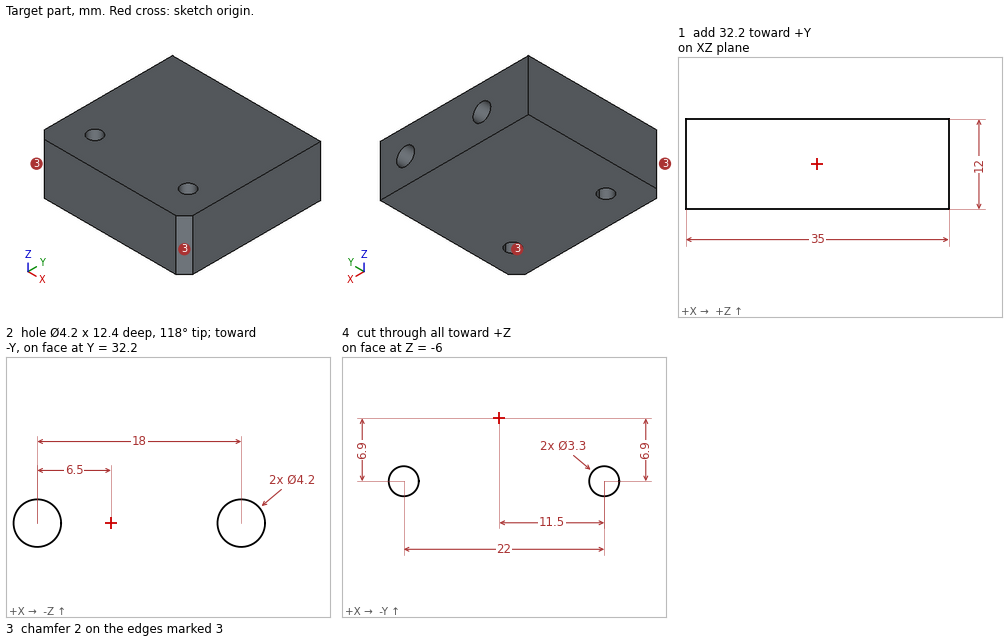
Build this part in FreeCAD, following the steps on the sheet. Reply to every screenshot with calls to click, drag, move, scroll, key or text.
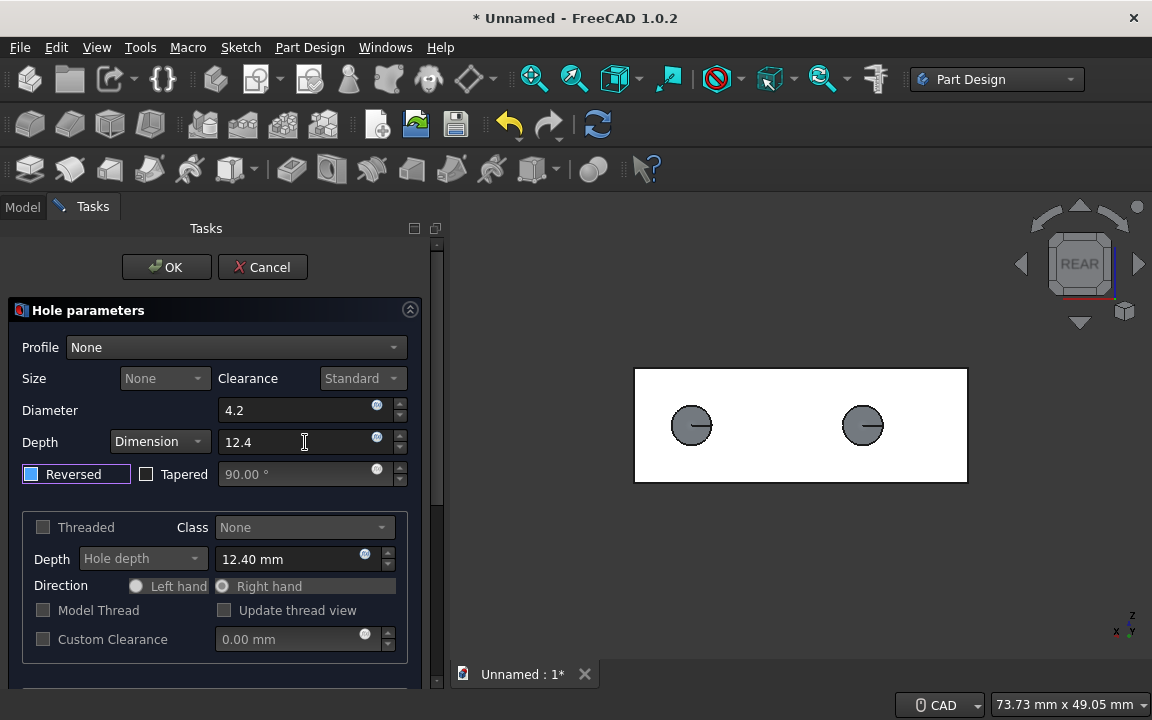
click(167, 267)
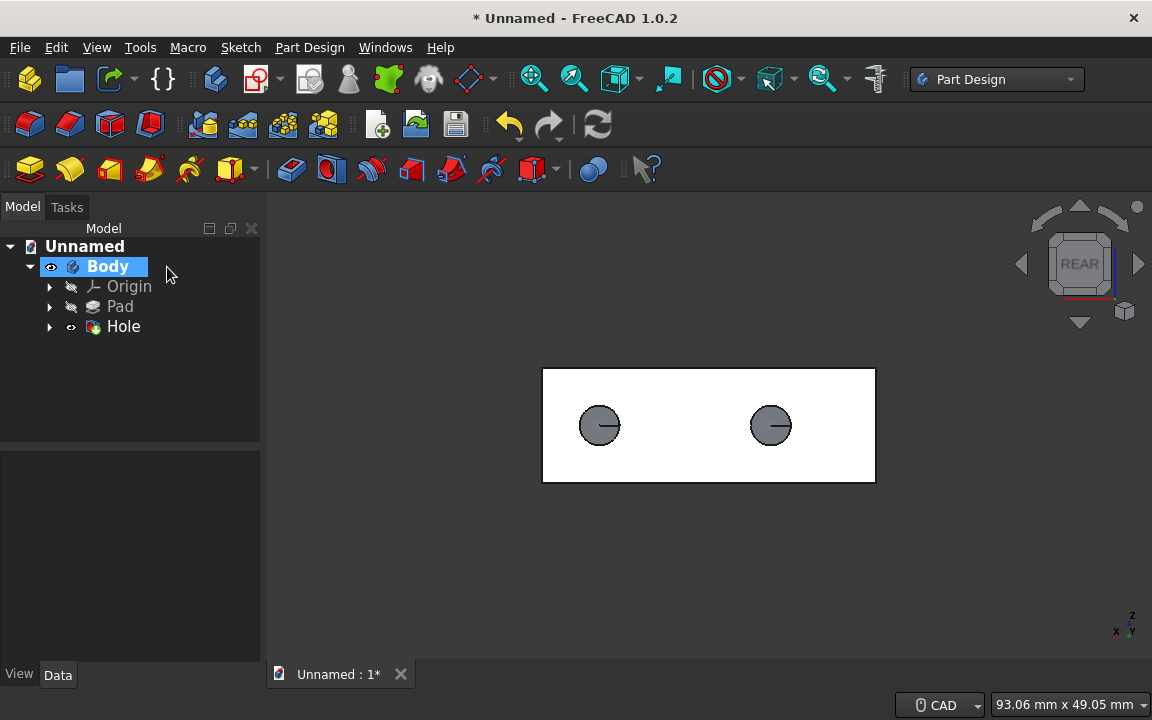
click(536, 80)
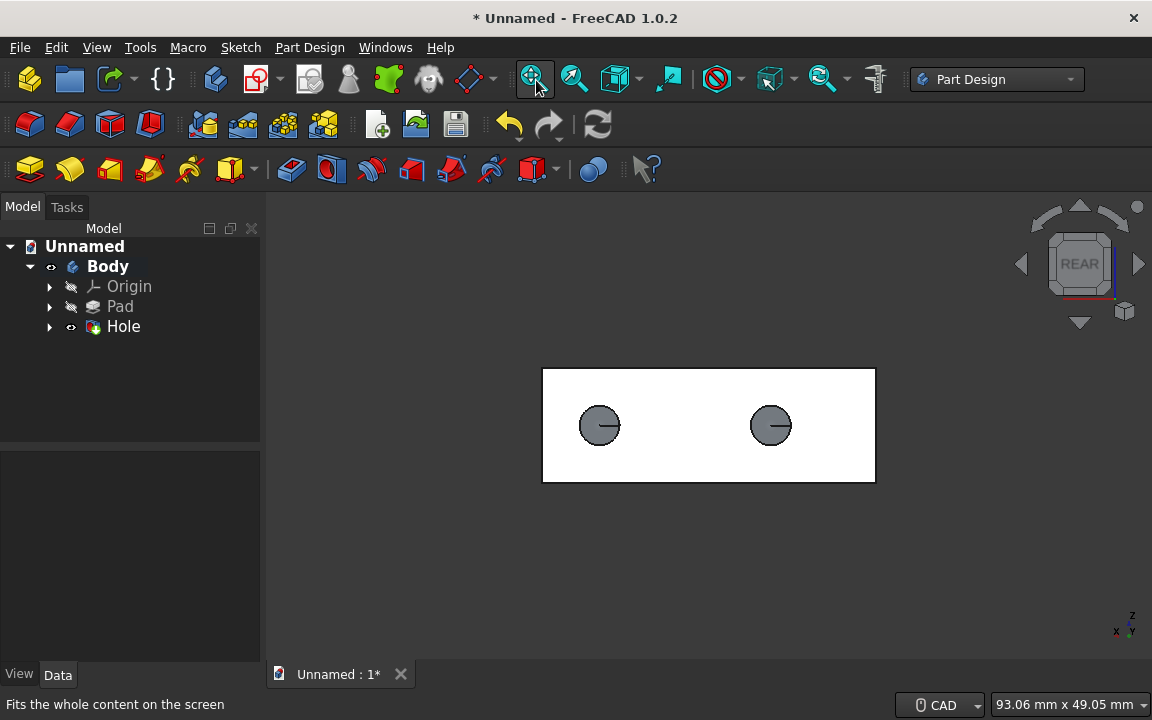
key(0)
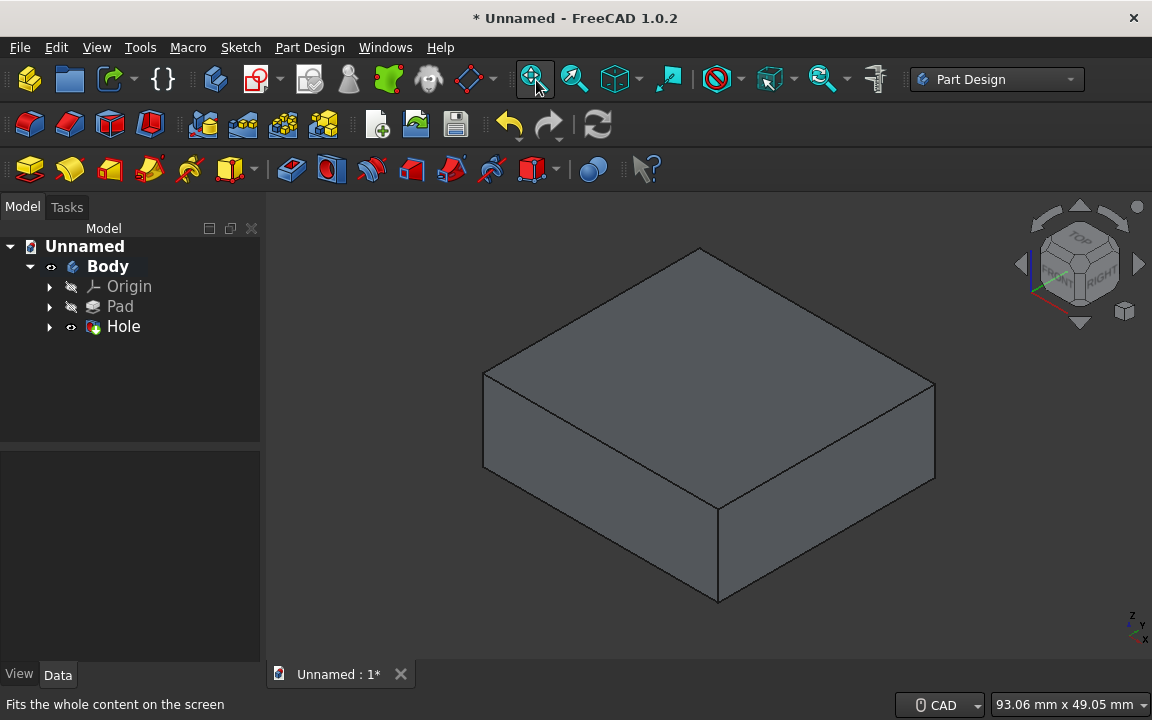
click(718, 555)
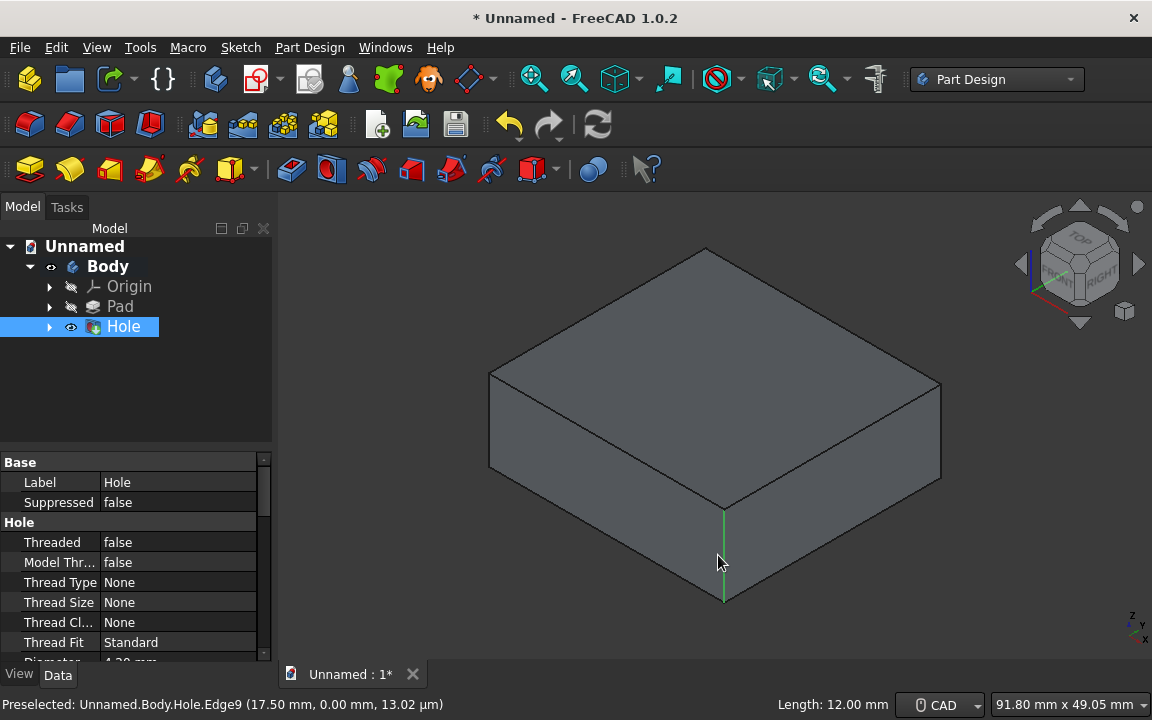
key(2)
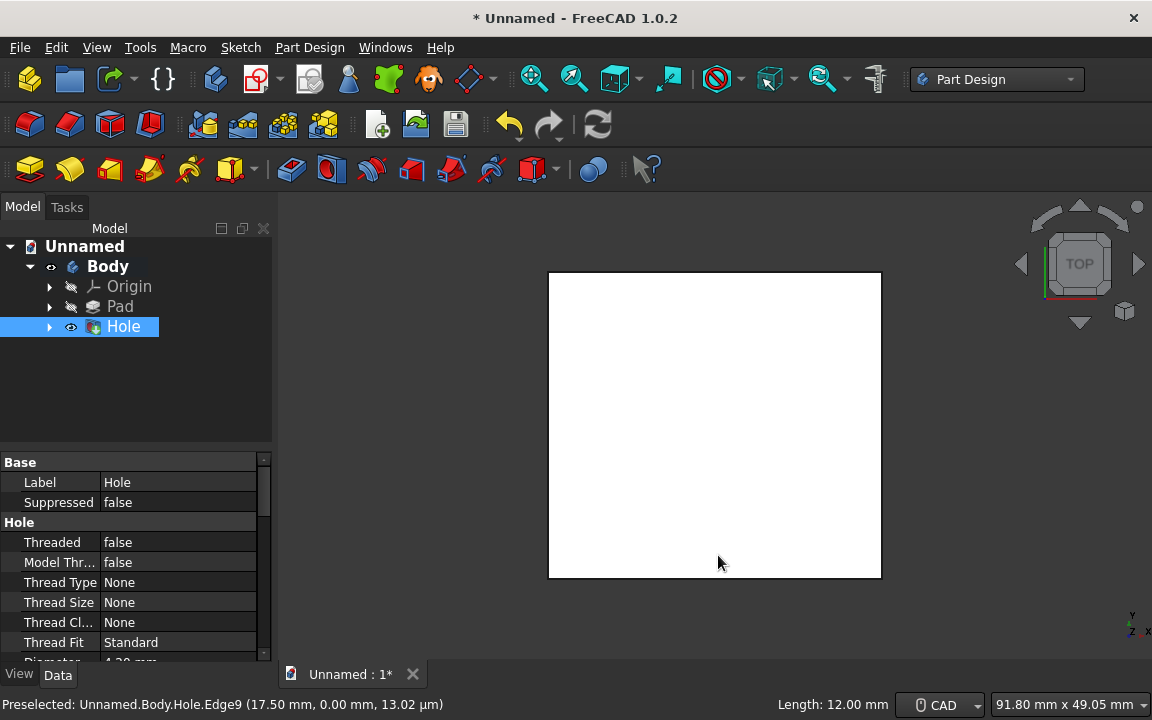
key(1)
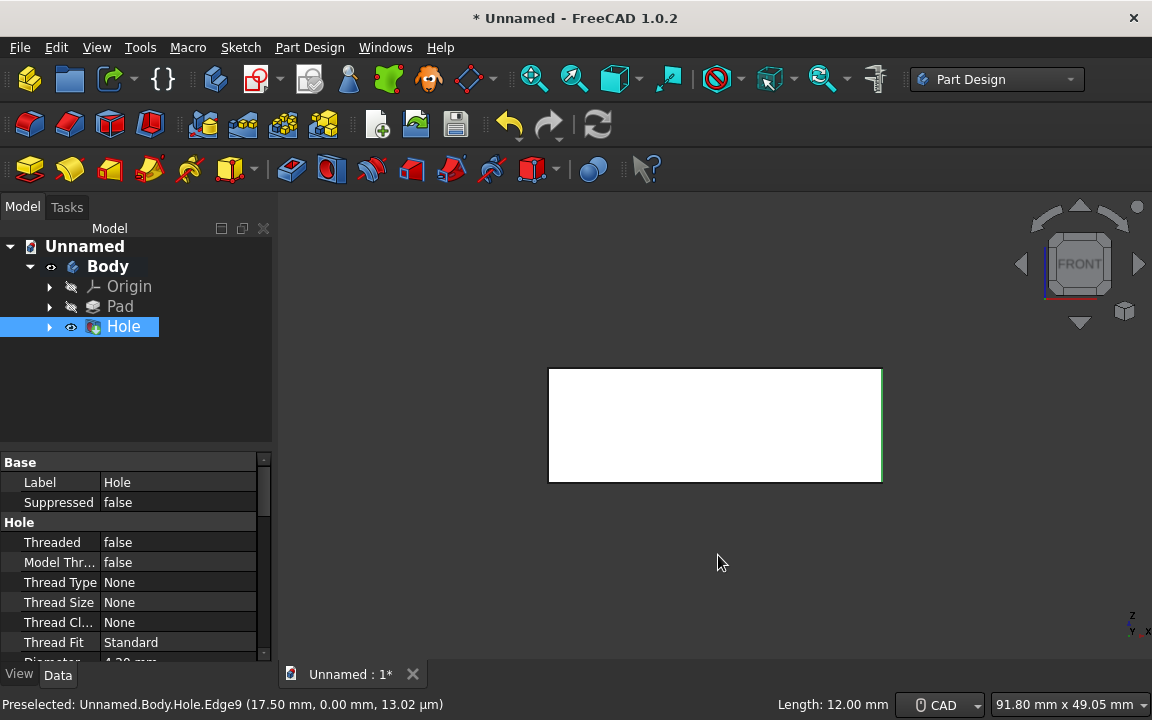
click(536, 80)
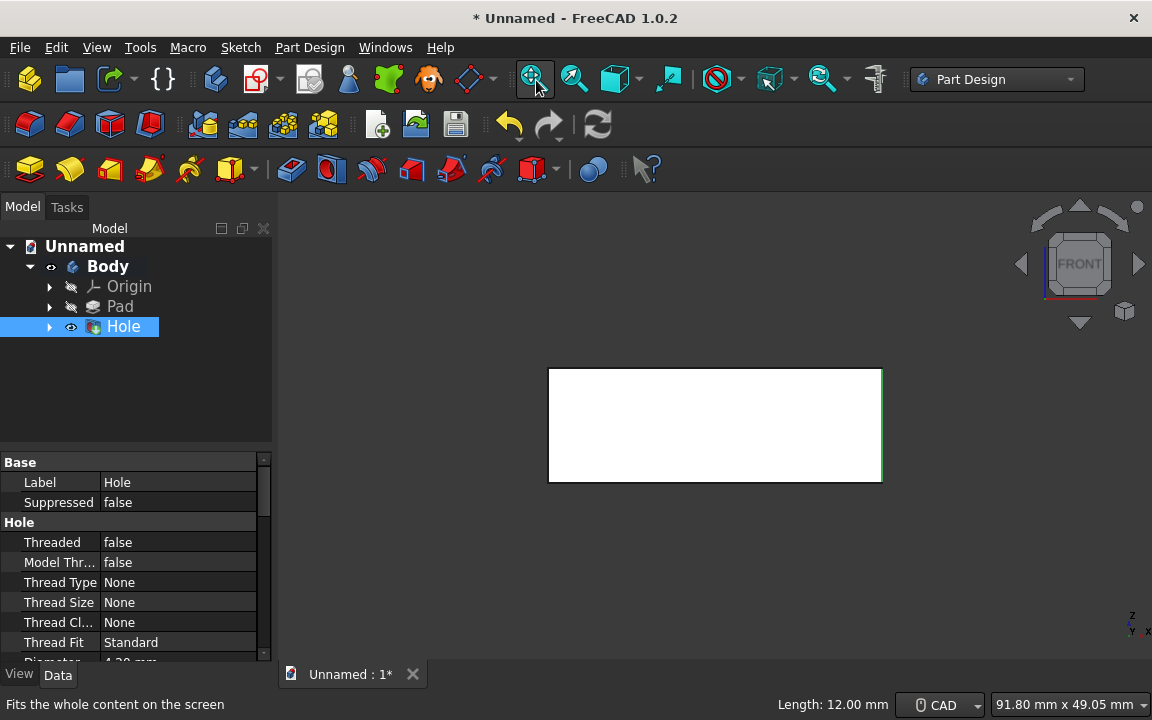
key(3)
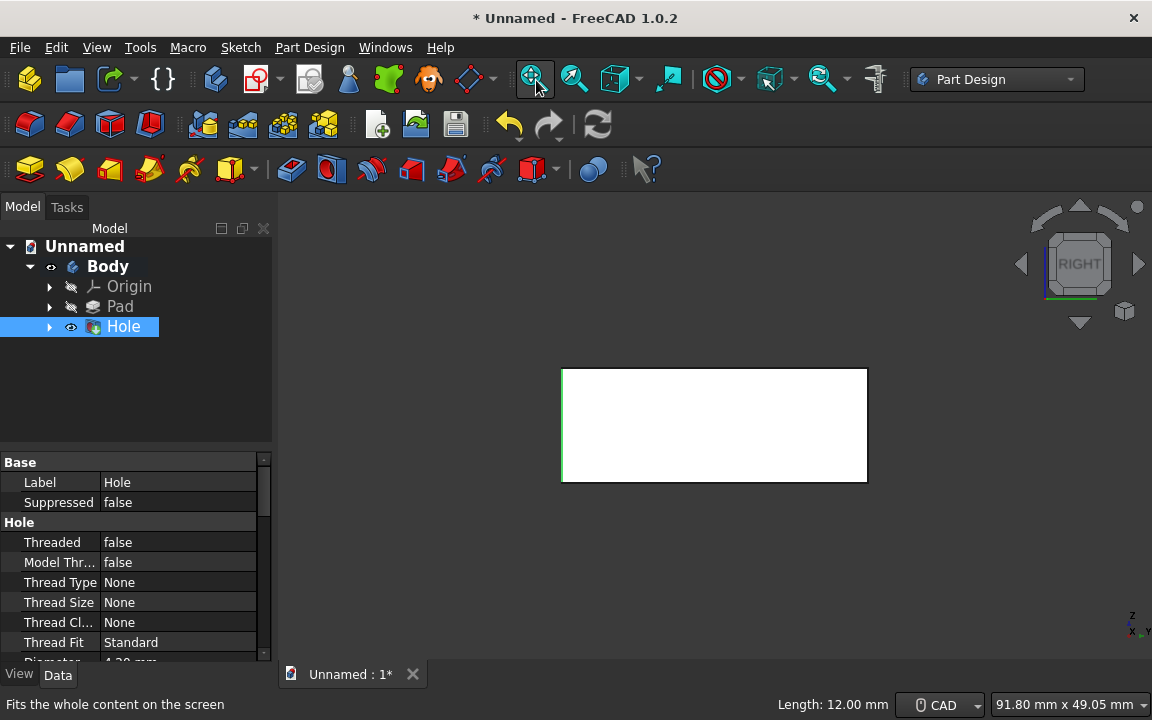
key(v)
key(f)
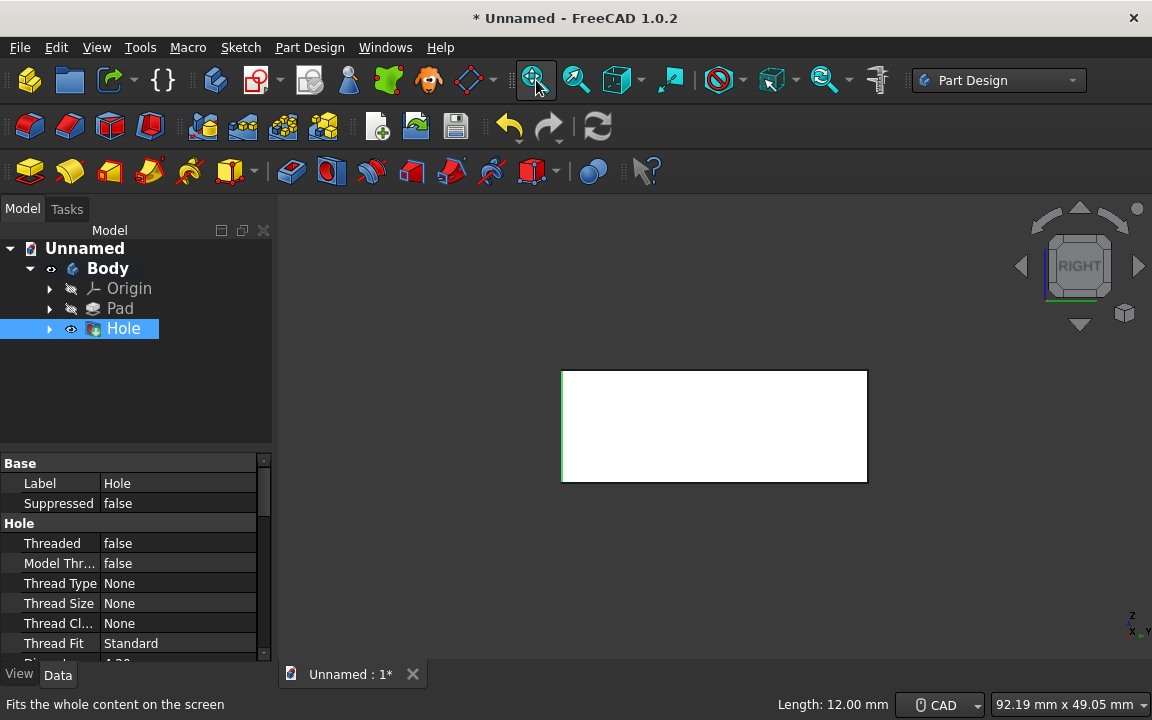
key(5)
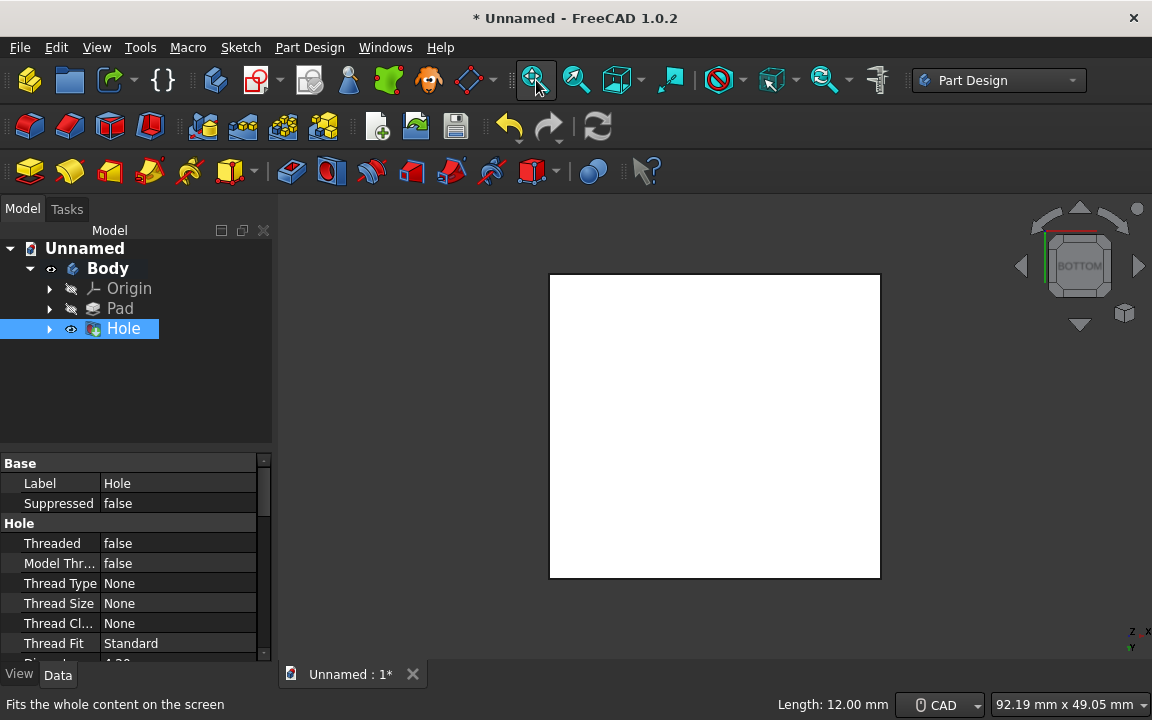
key(4)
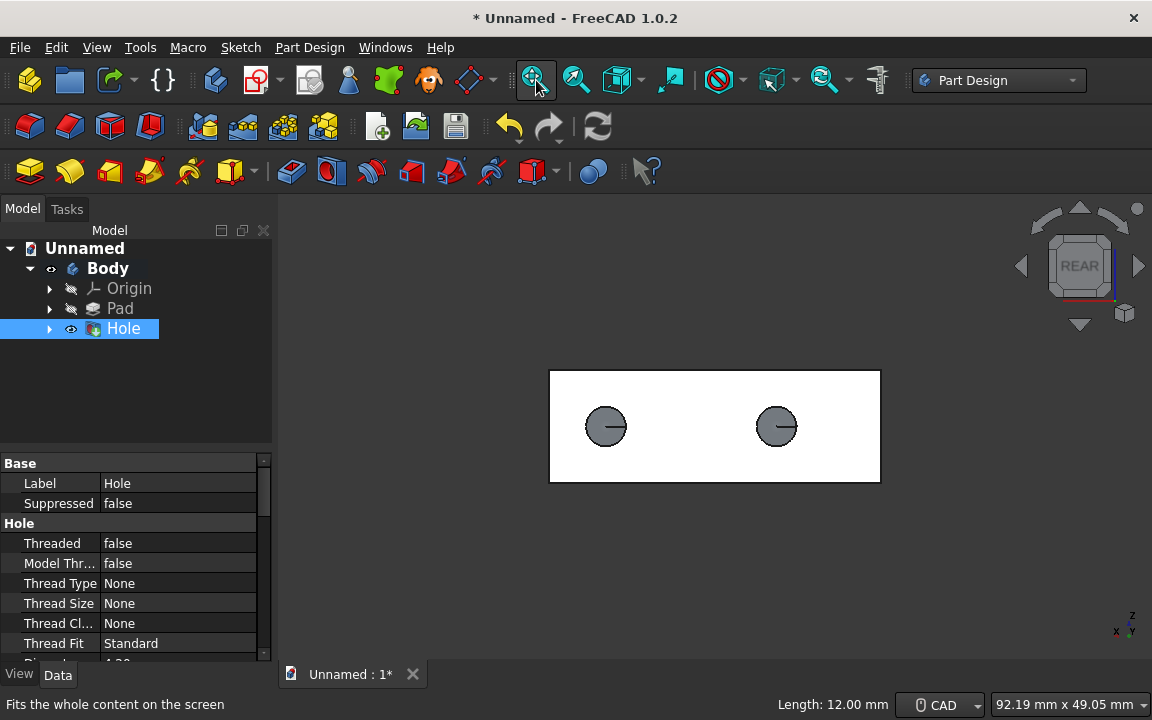
click(536, 80)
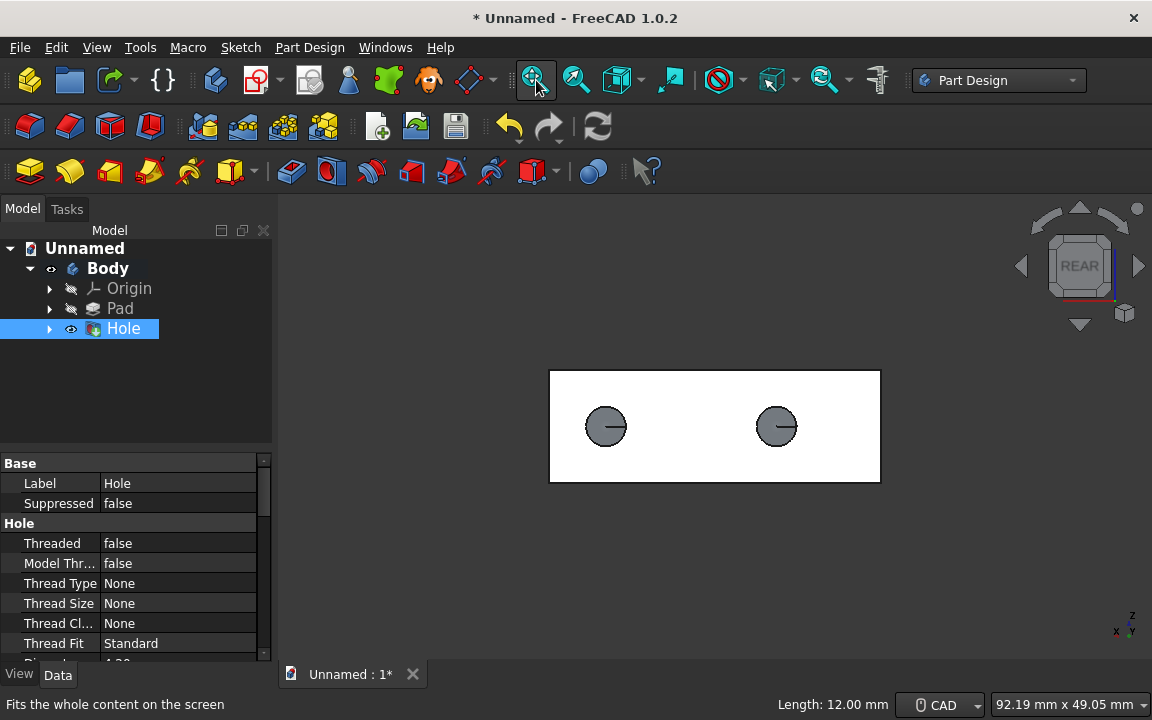
key(6)